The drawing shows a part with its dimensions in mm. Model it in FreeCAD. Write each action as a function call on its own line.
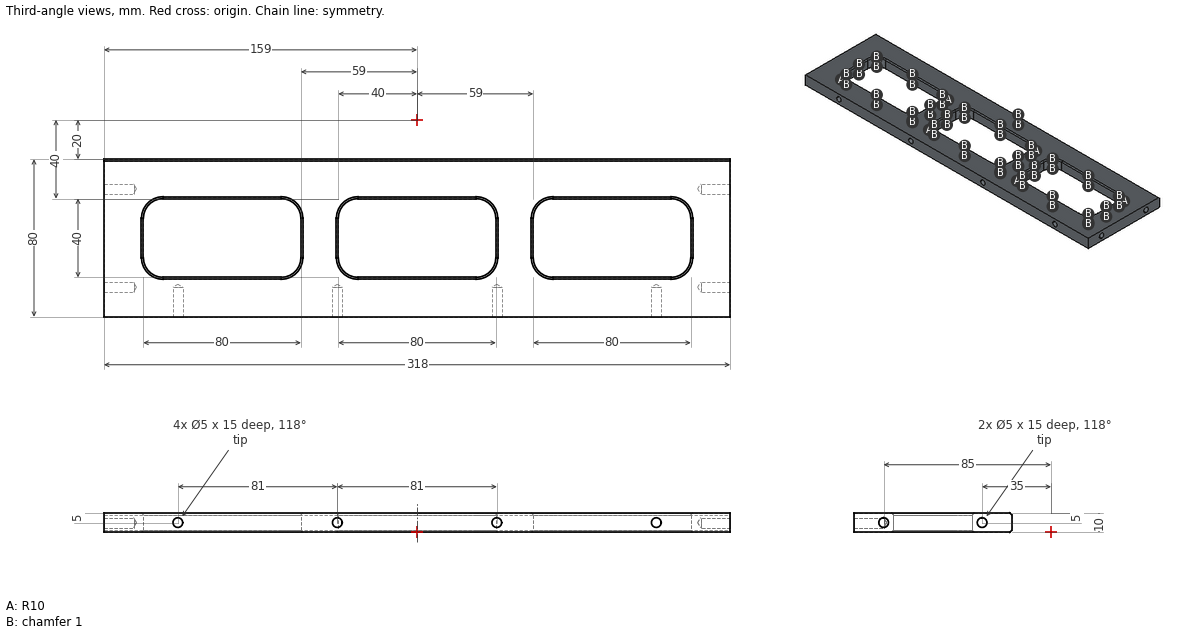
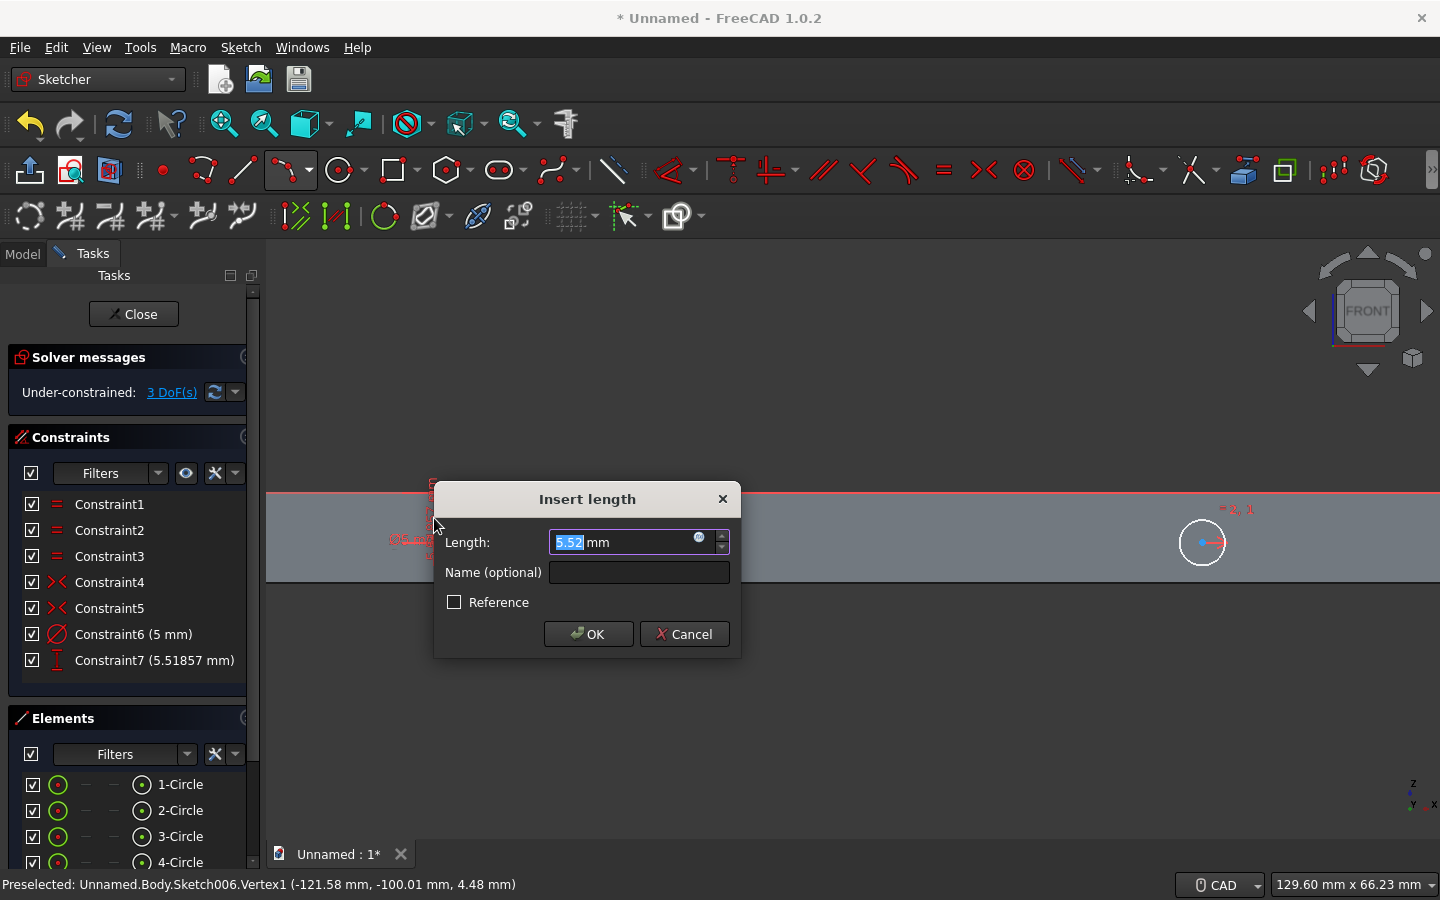
text(5)
key(Return)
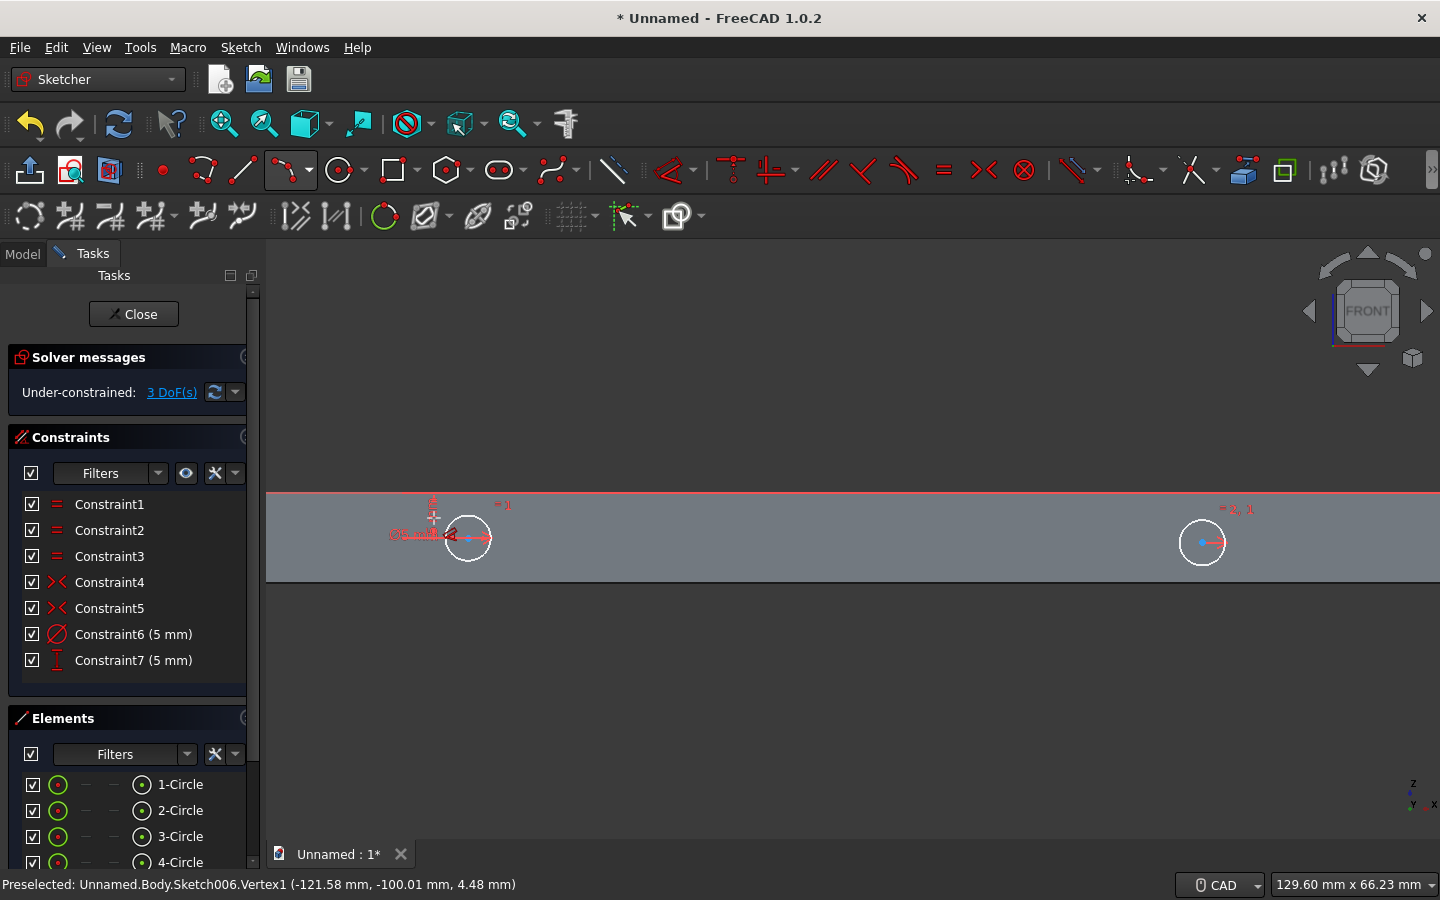
click(1202, 543)
click(1168, 518)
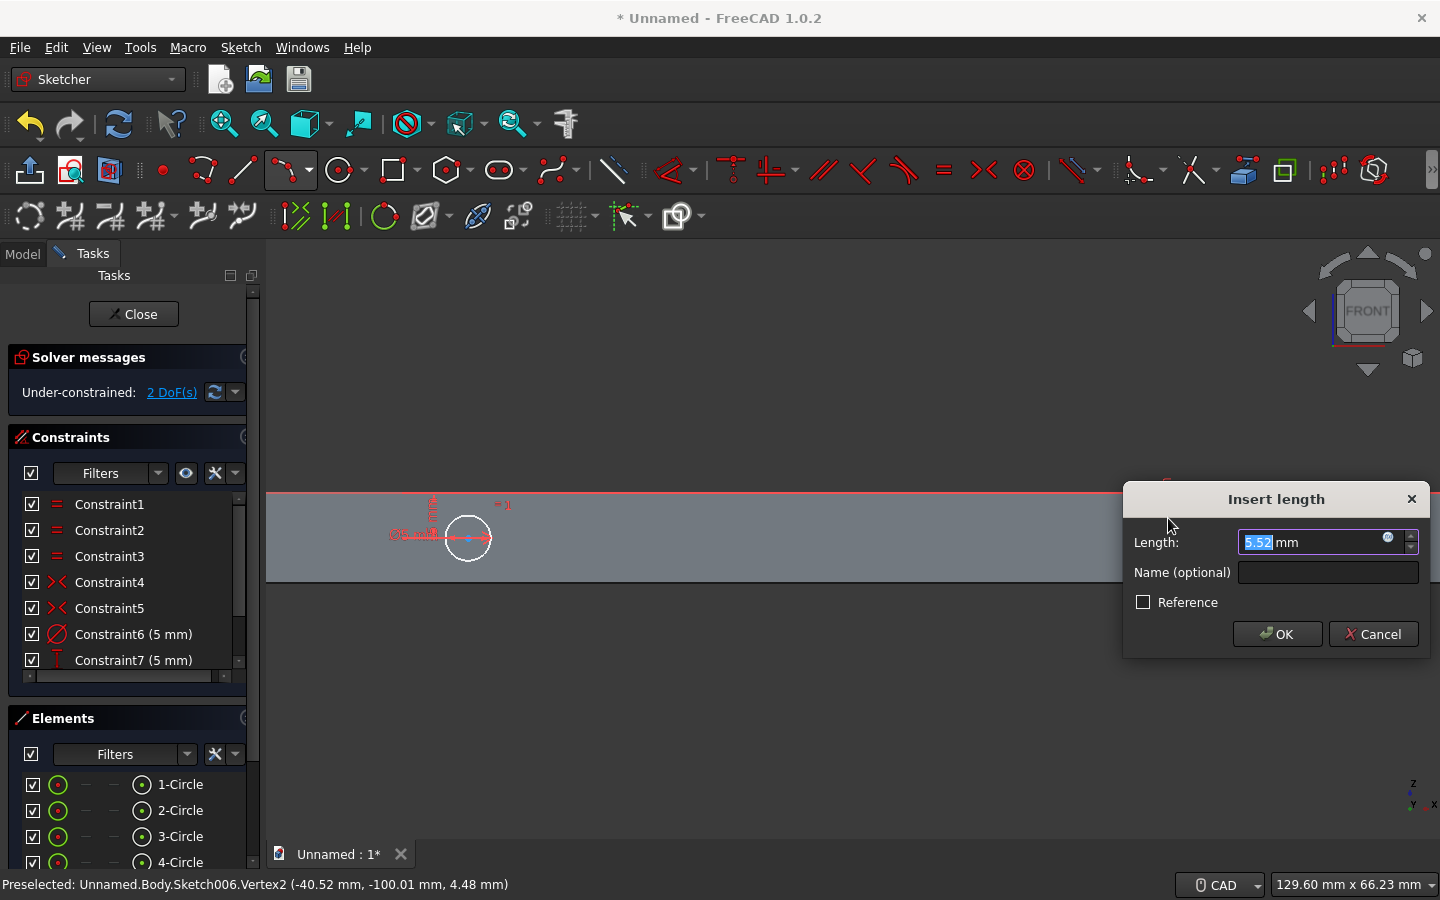
text(5)
key(Return)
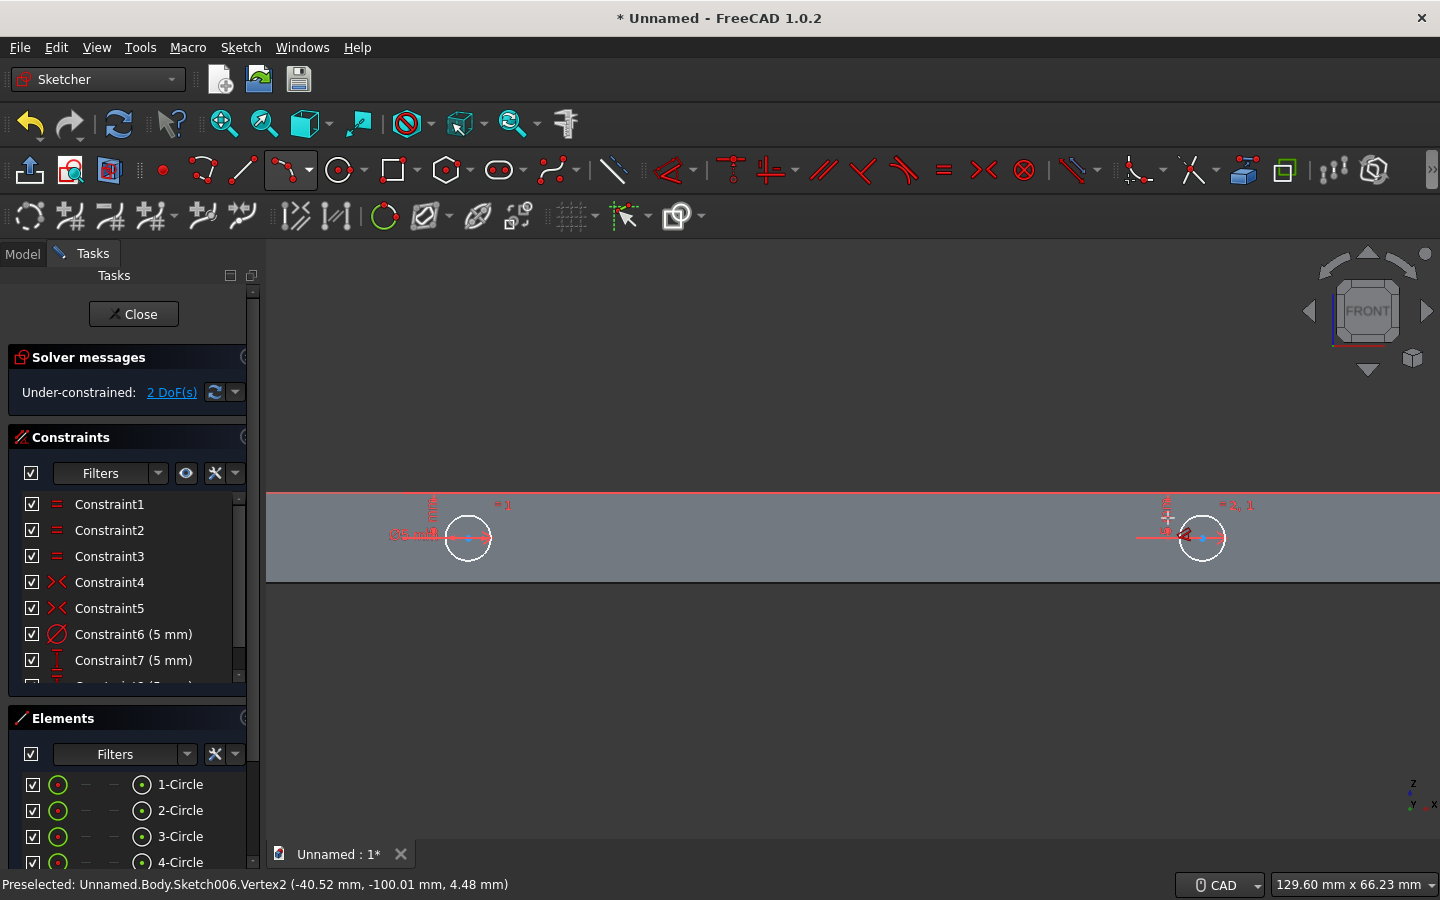
click(468, 538)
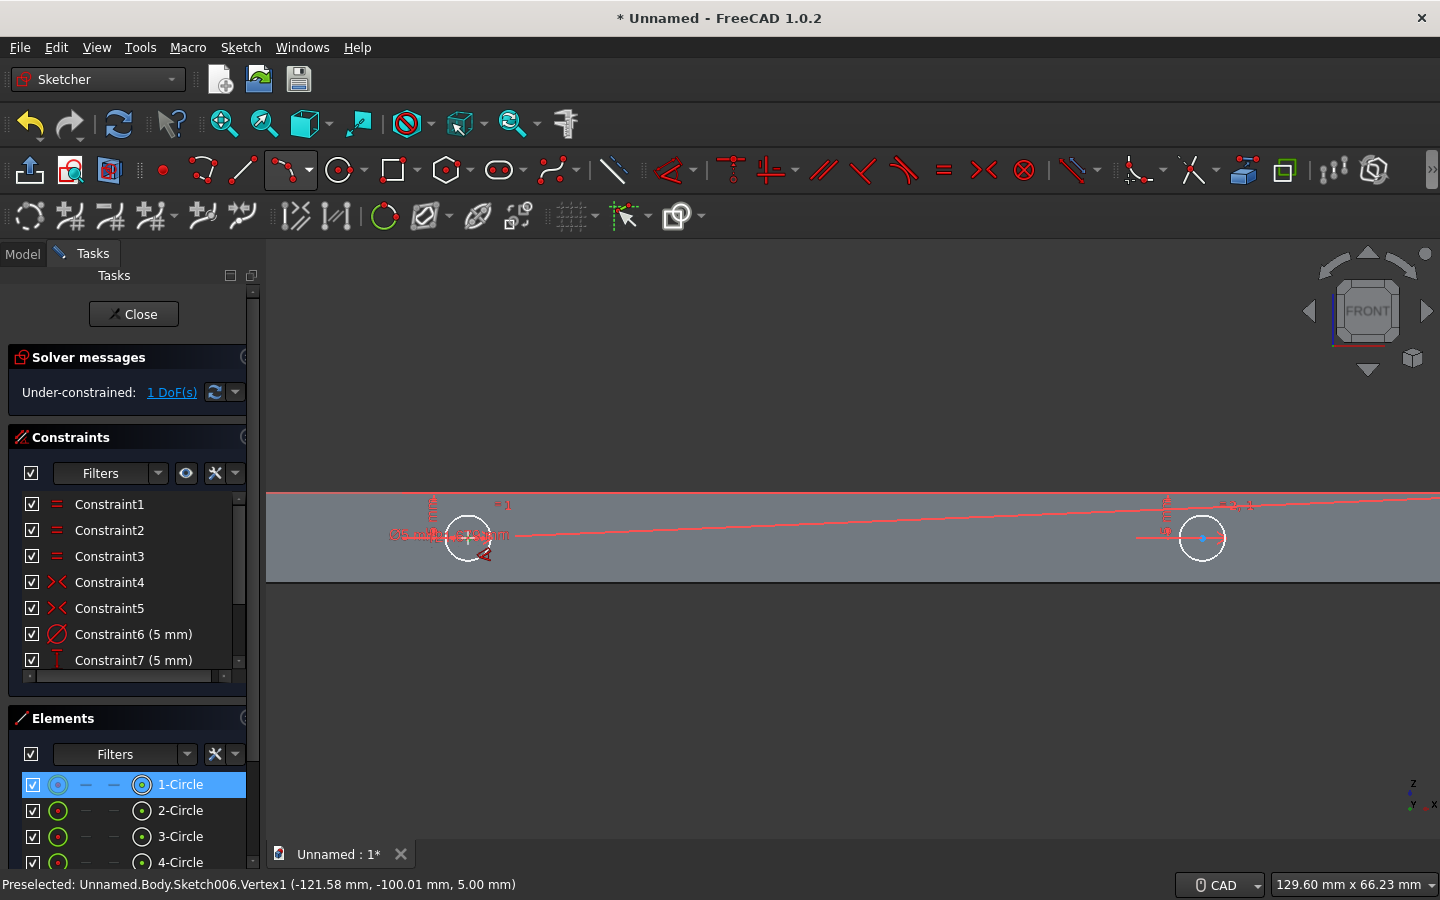
click(1202, 538)
click(835, 572)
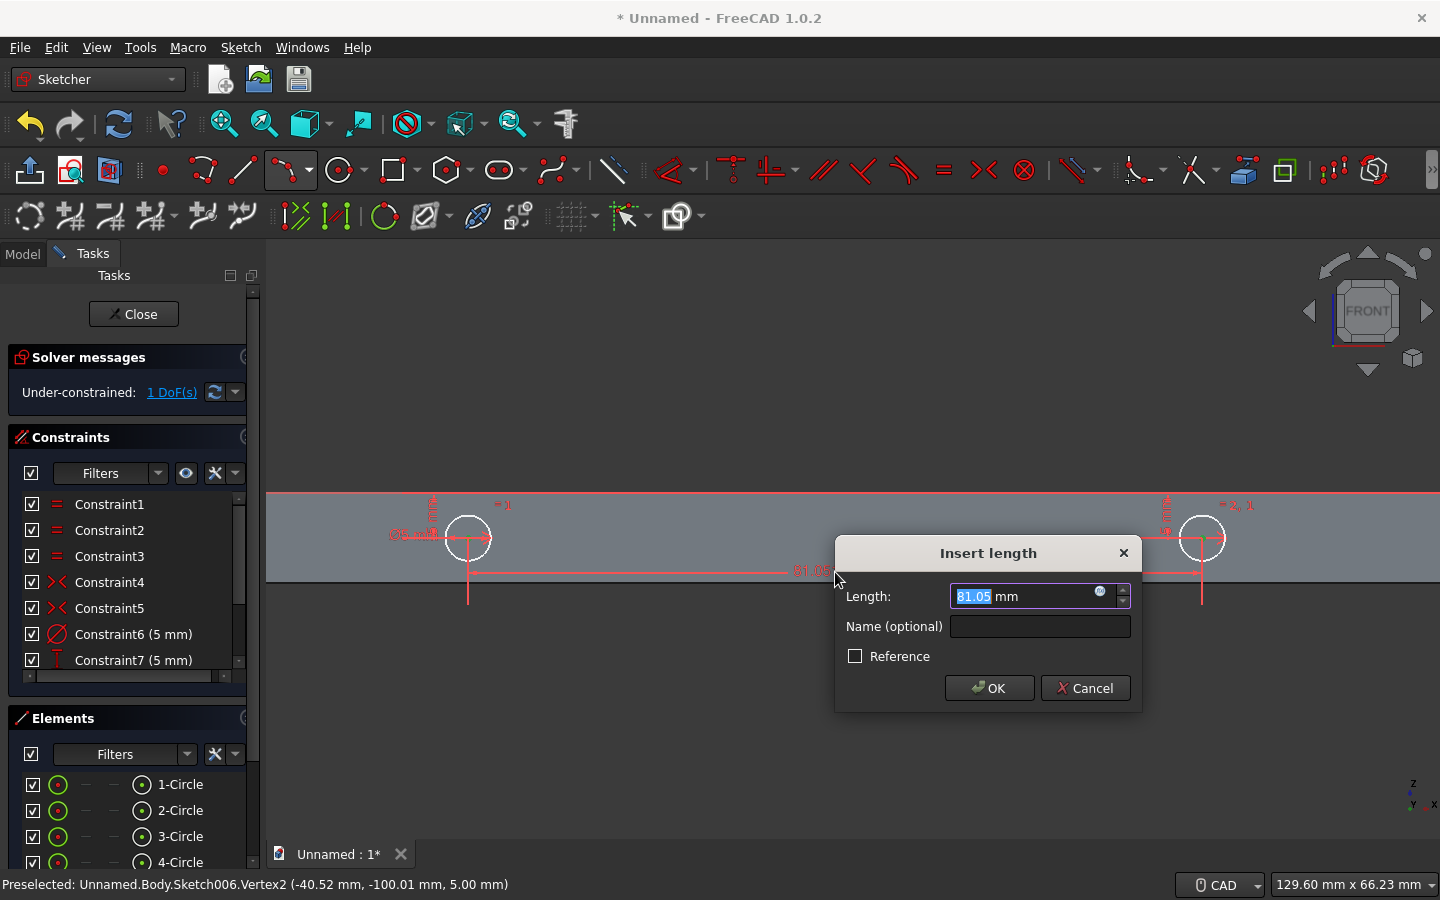
text(81)
key(Return)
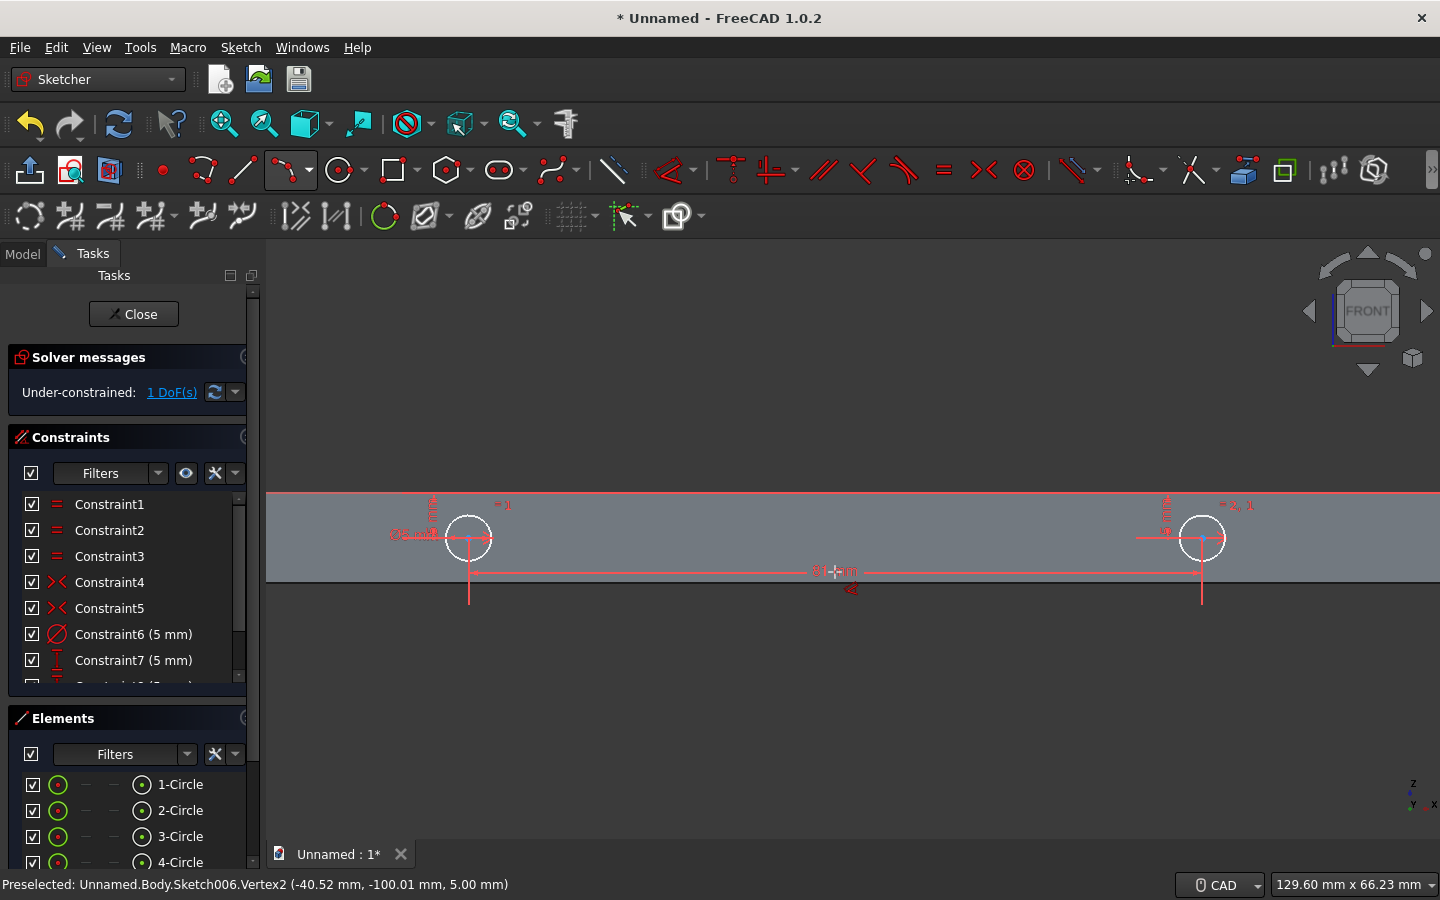
click(1202, 538)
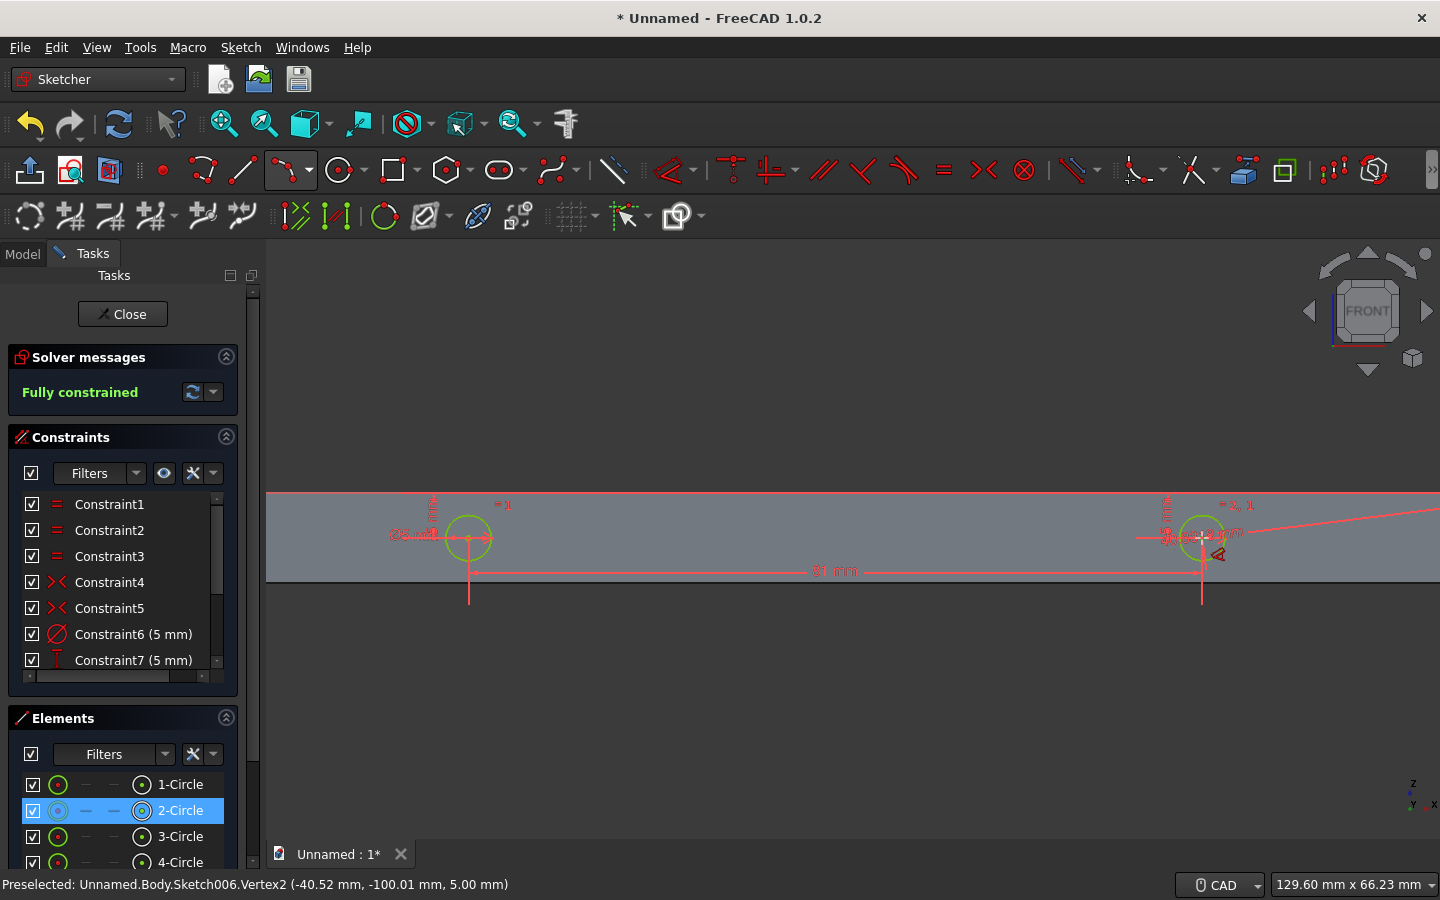
scroll(446, 544, down, 6)